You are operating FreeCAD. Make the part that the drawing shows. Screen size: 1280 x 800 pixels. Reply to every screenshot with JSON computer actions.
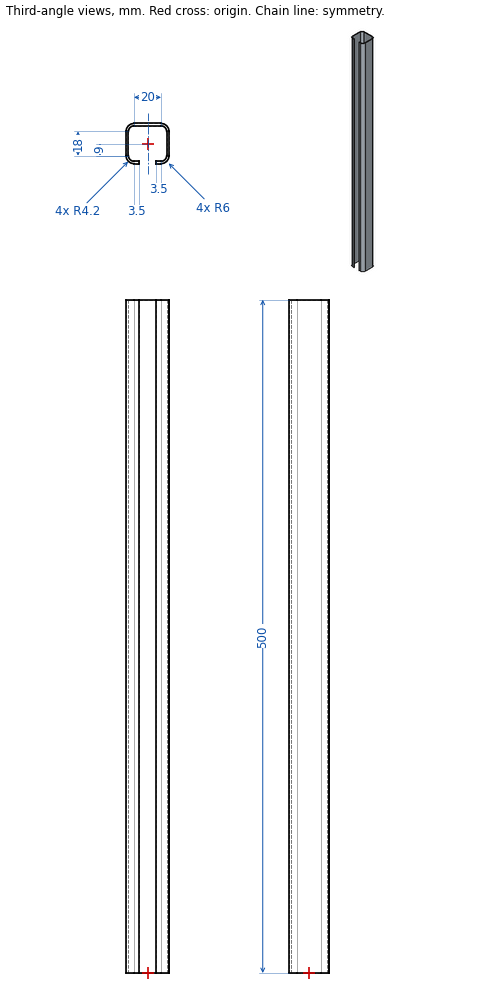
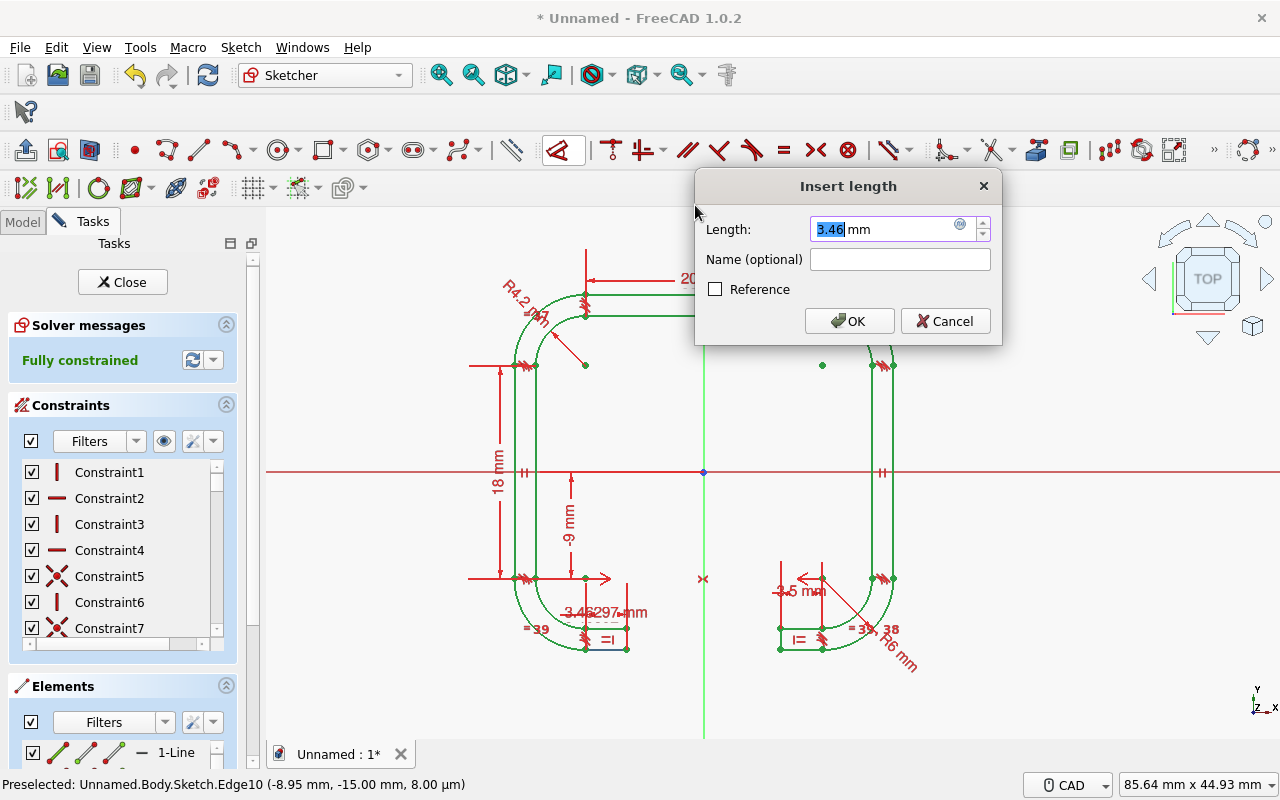
{"action": "type", "text": "3.5"}
{"action": "key", "text": "Return"}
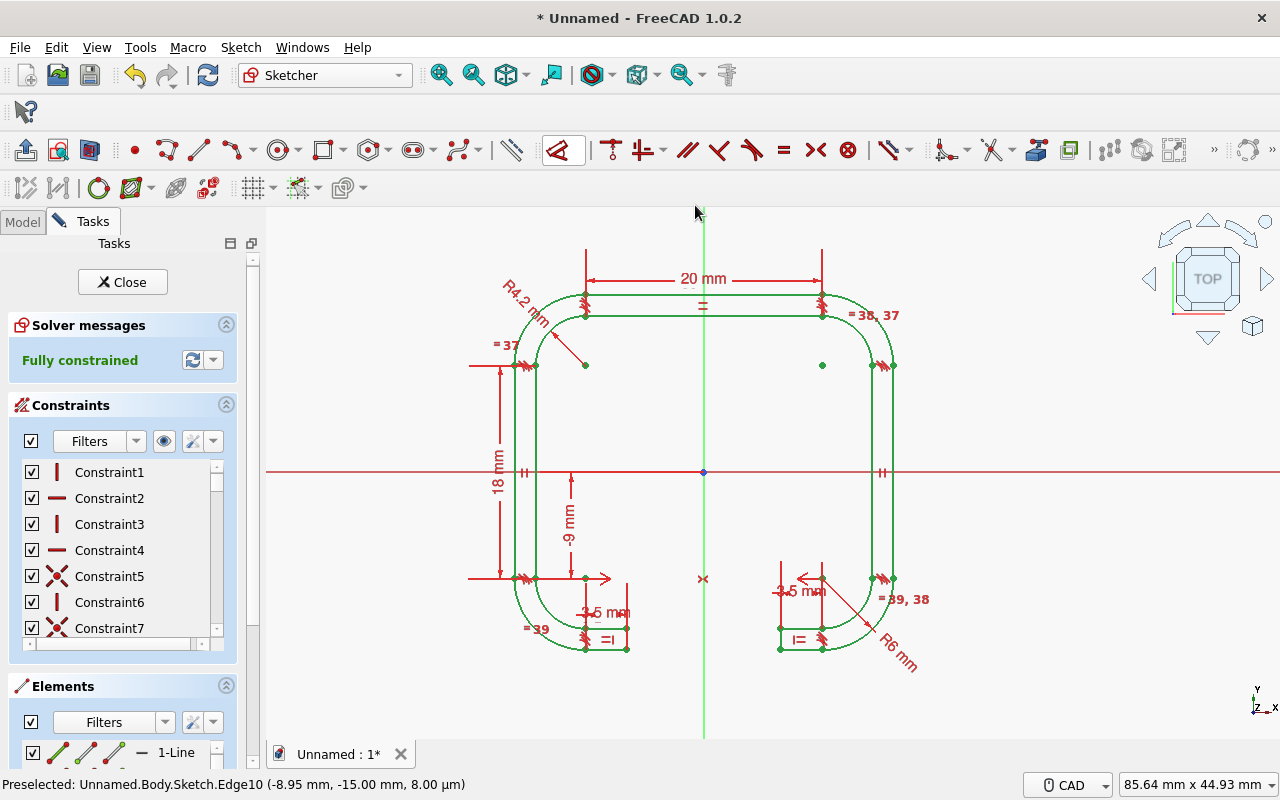
{"action": "left_click", "coordinate": [123, 282]}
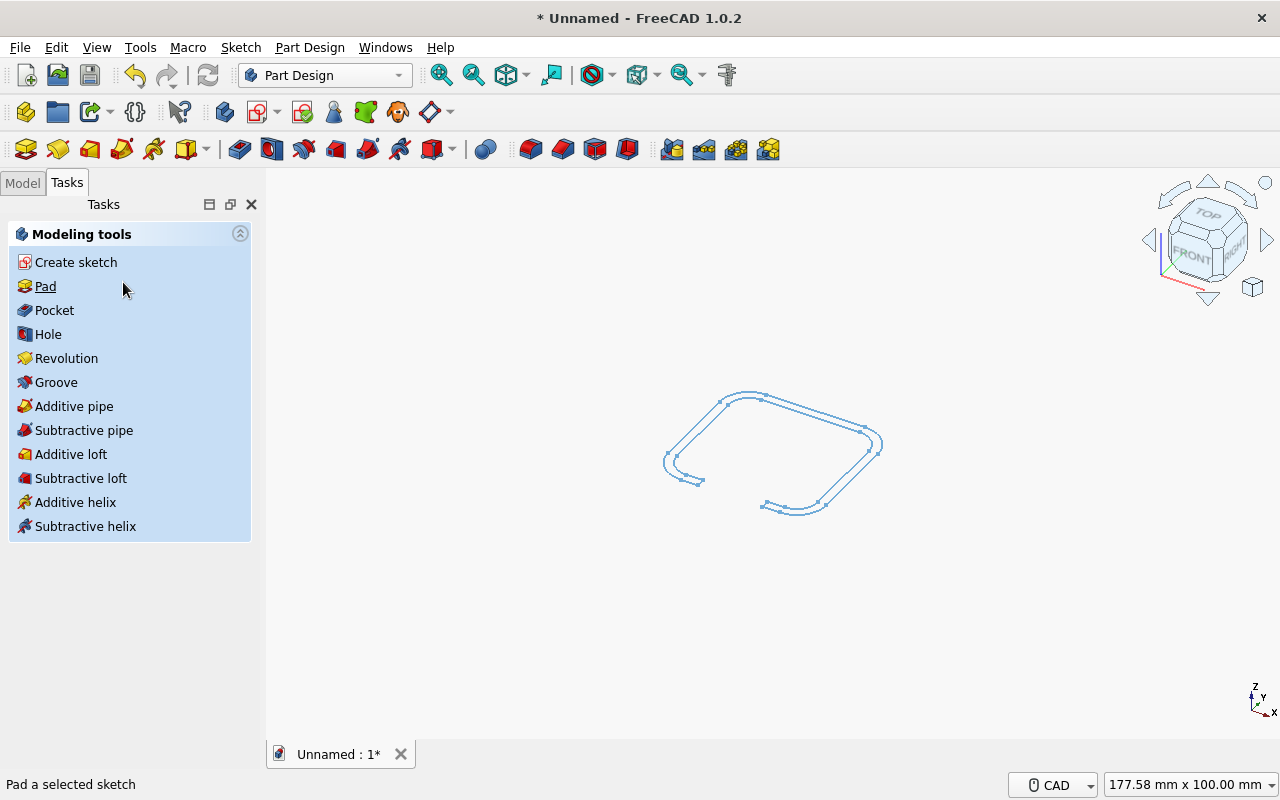
{"action": "left_click", "coordinate": [26, 150]}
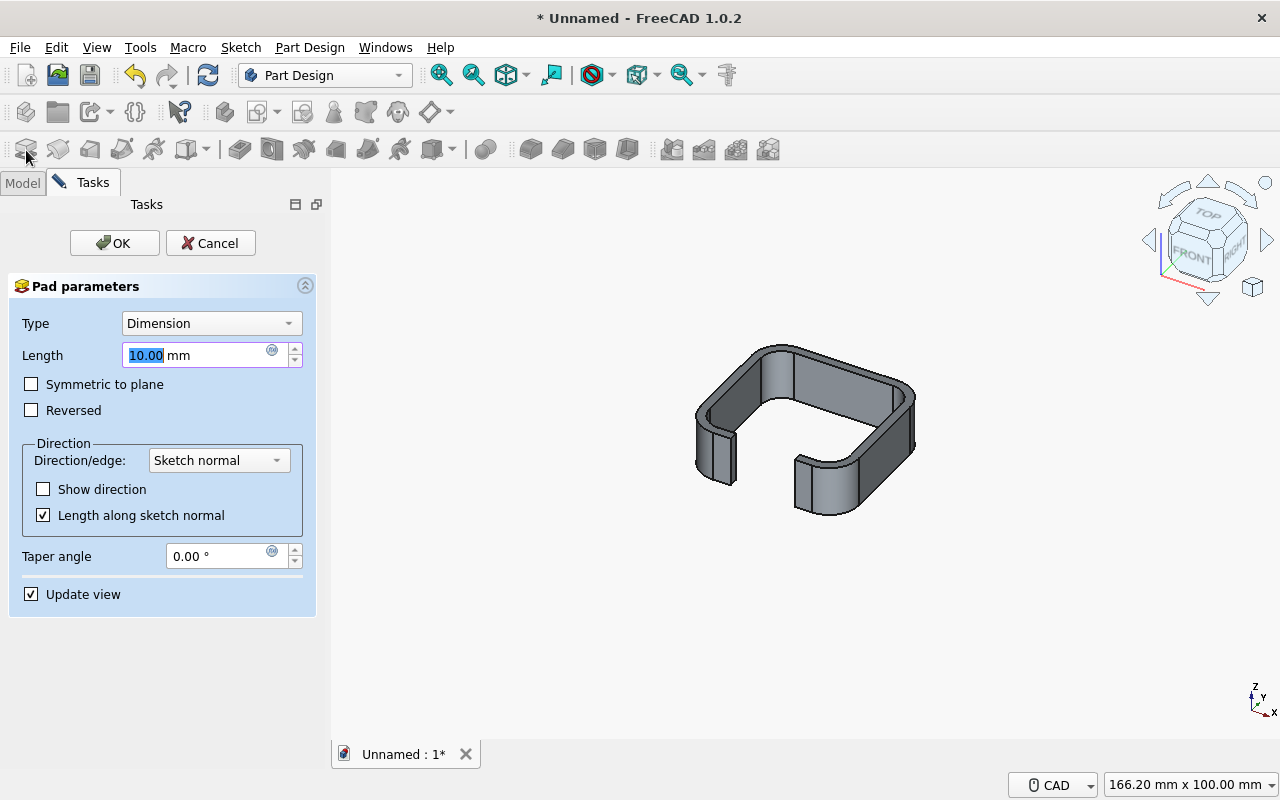
{"action": "type", "text": "500"}
{"action": "key", "text": "Tab"}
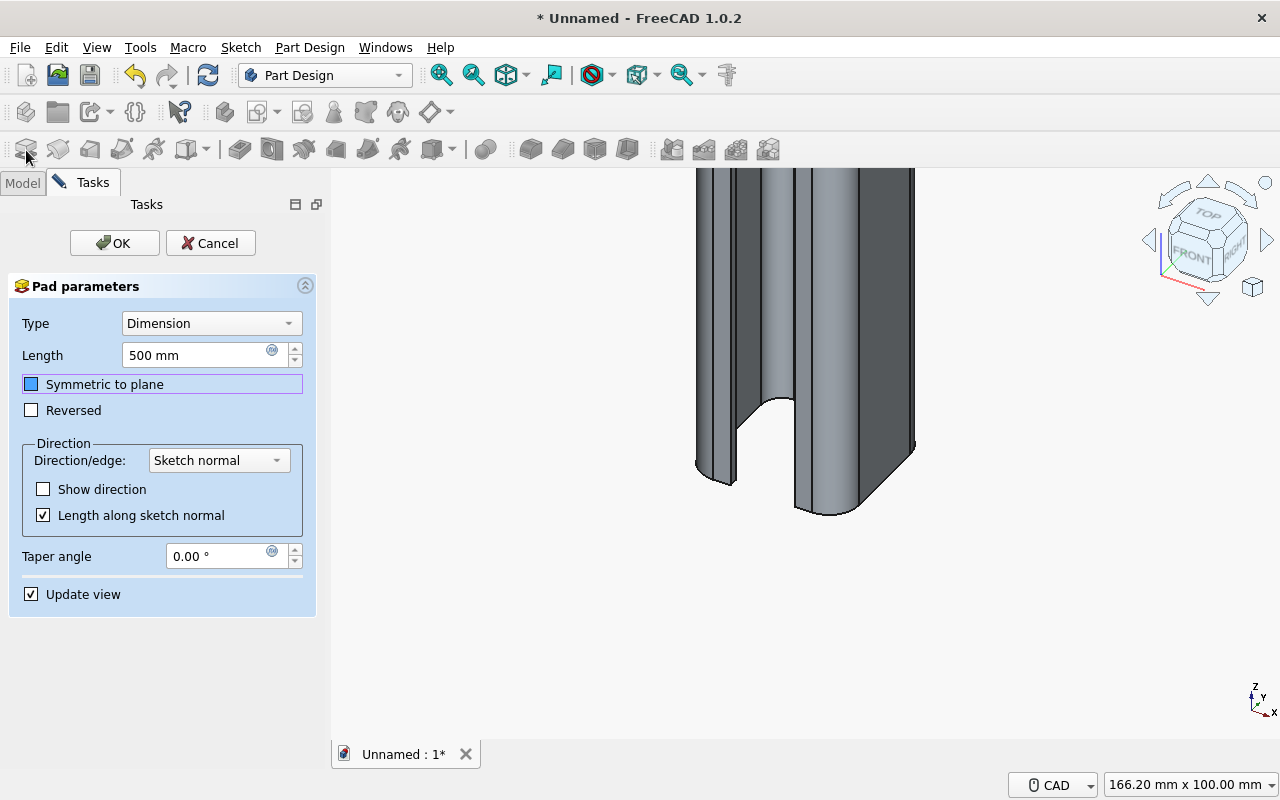
{"action": "left_click", "coordinate": [115, 243]}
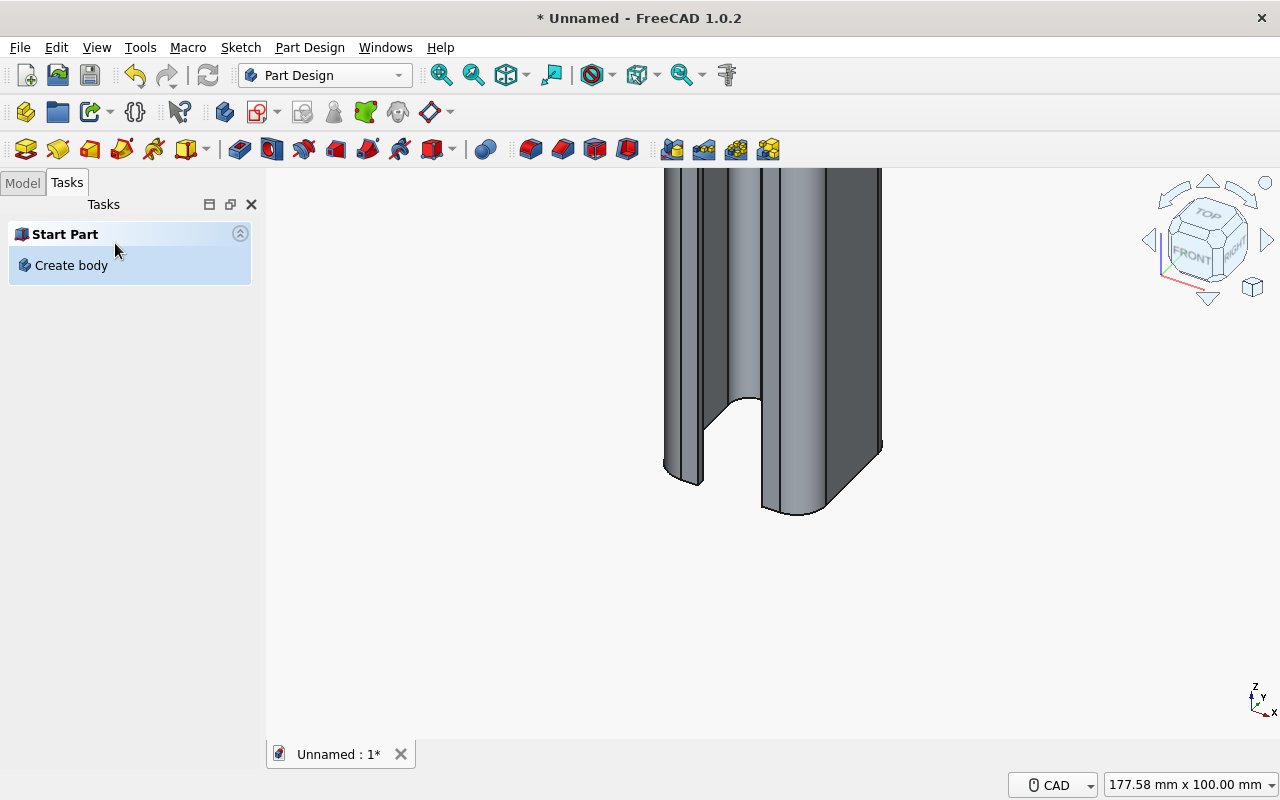
{"action": "key", "text": "0"}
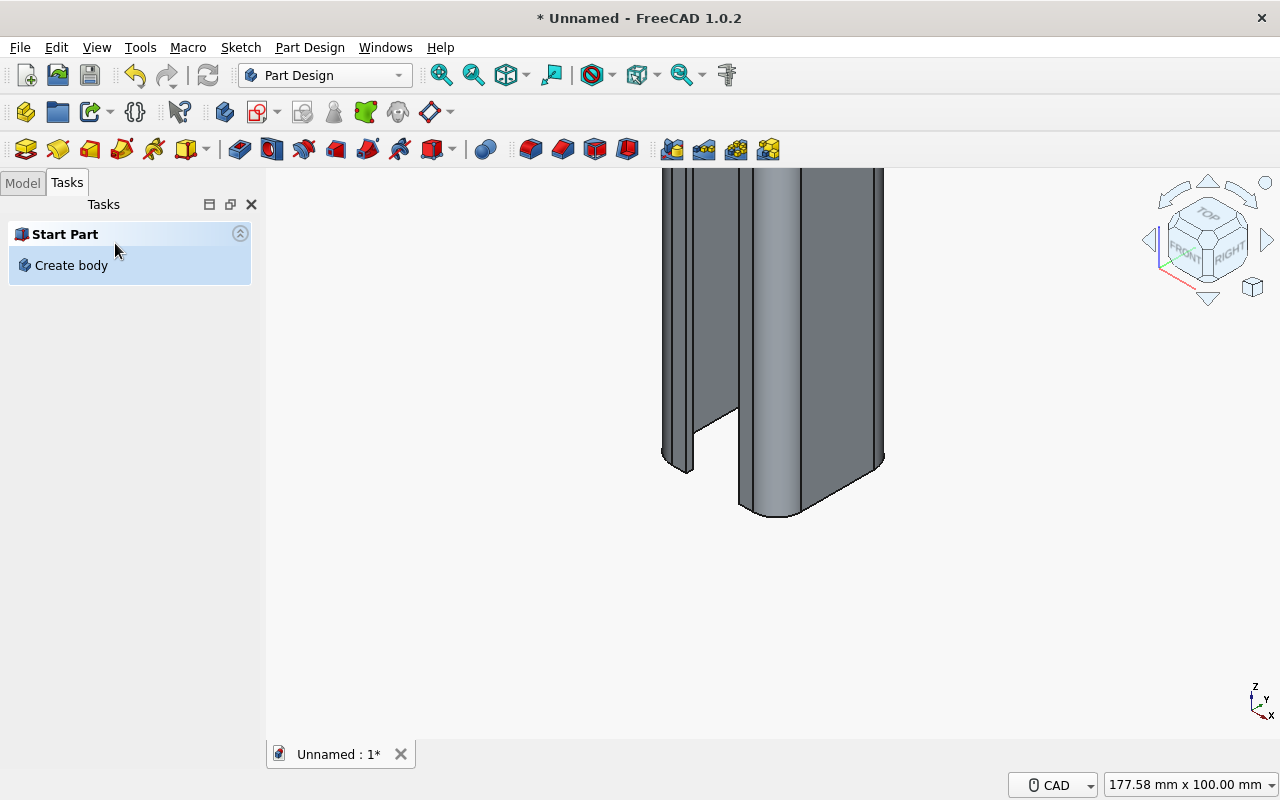
{"action": "left_click", "coordinate": [442, 76]}